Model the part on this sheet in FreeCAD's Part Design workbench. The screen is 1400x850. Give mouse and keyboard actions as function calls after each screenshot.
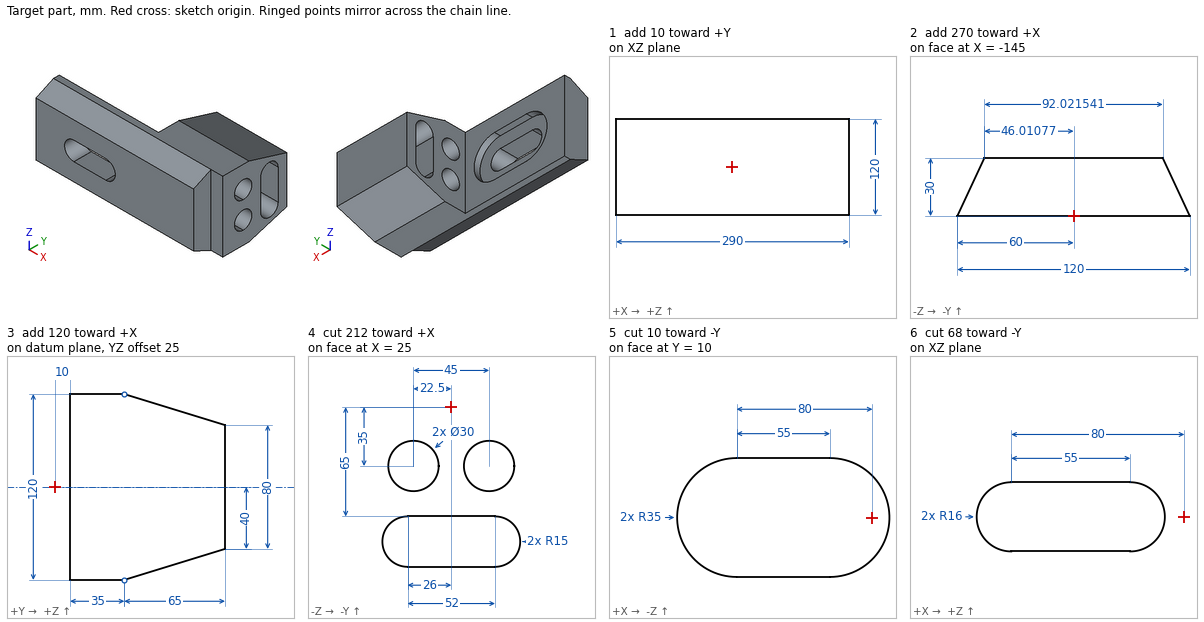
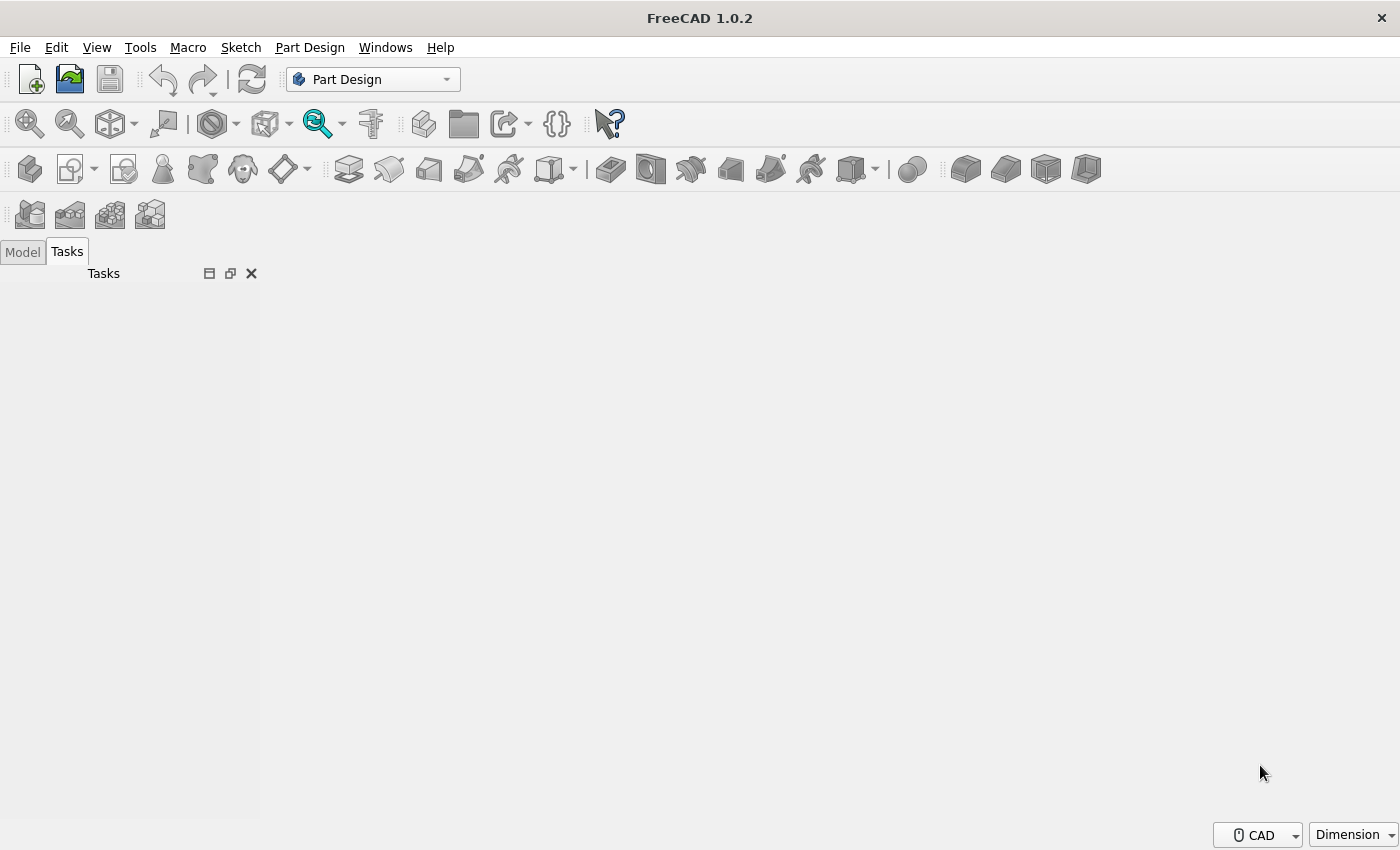
key(ctrl+n)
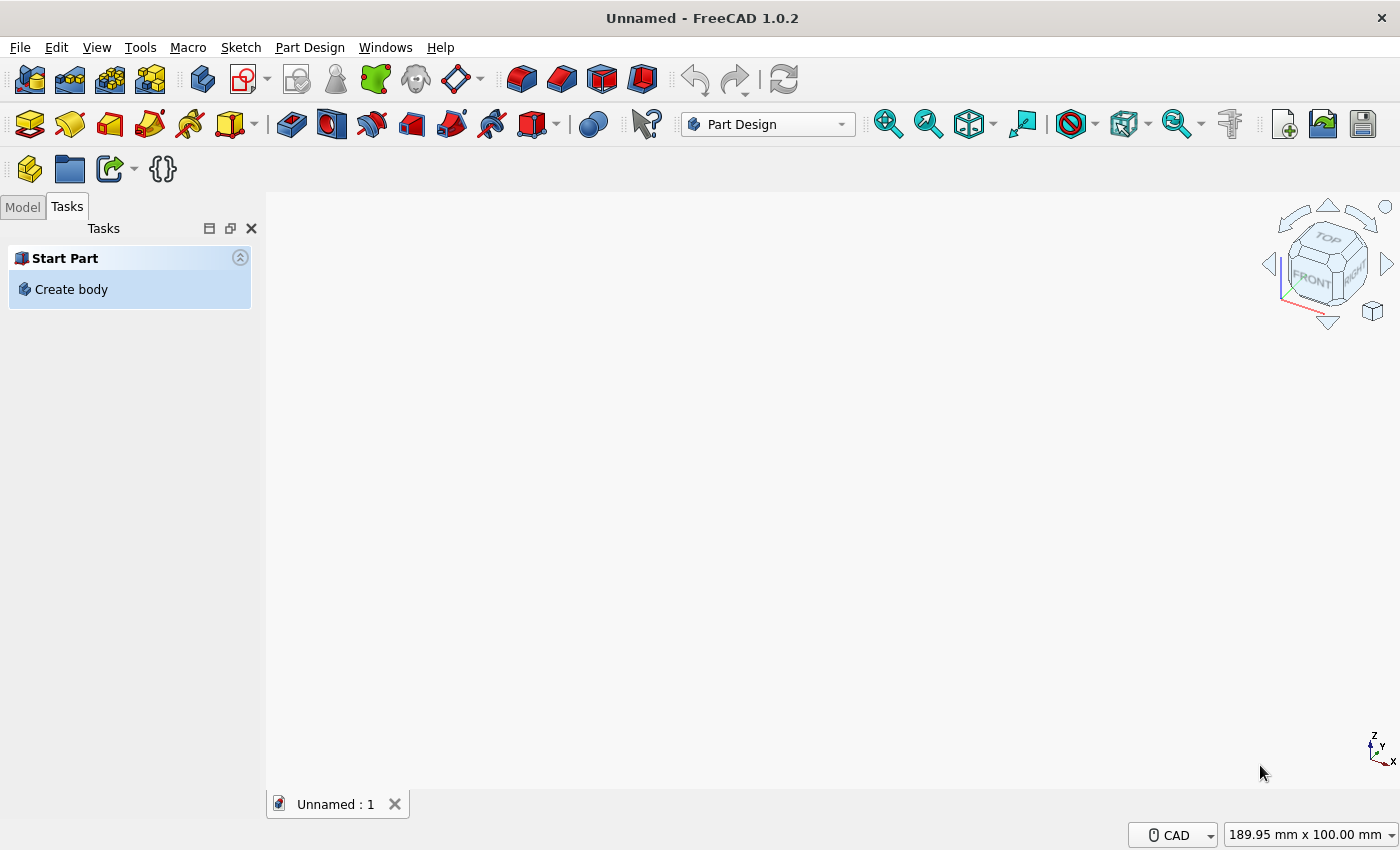
click(244, 80)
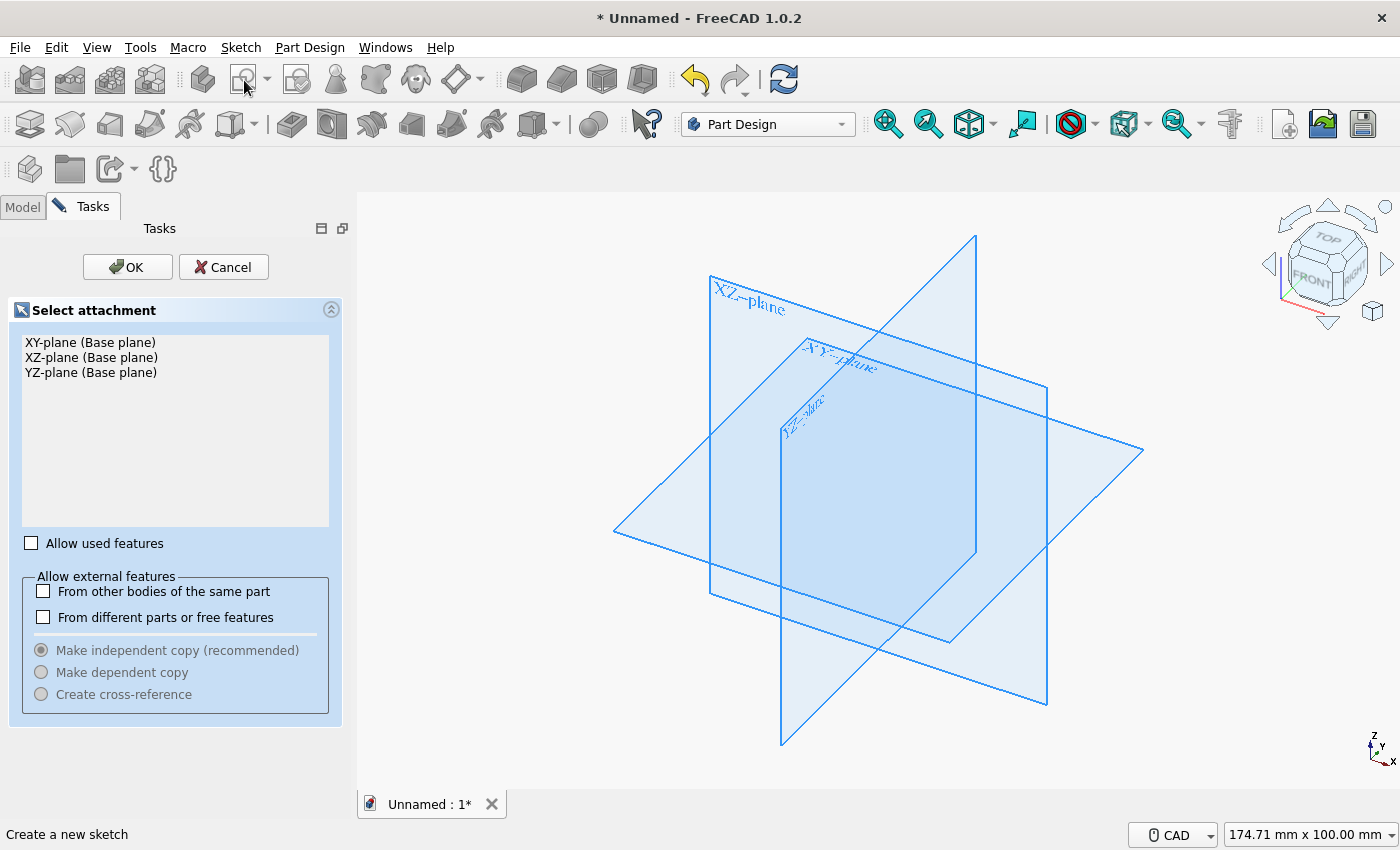
click(82, 358)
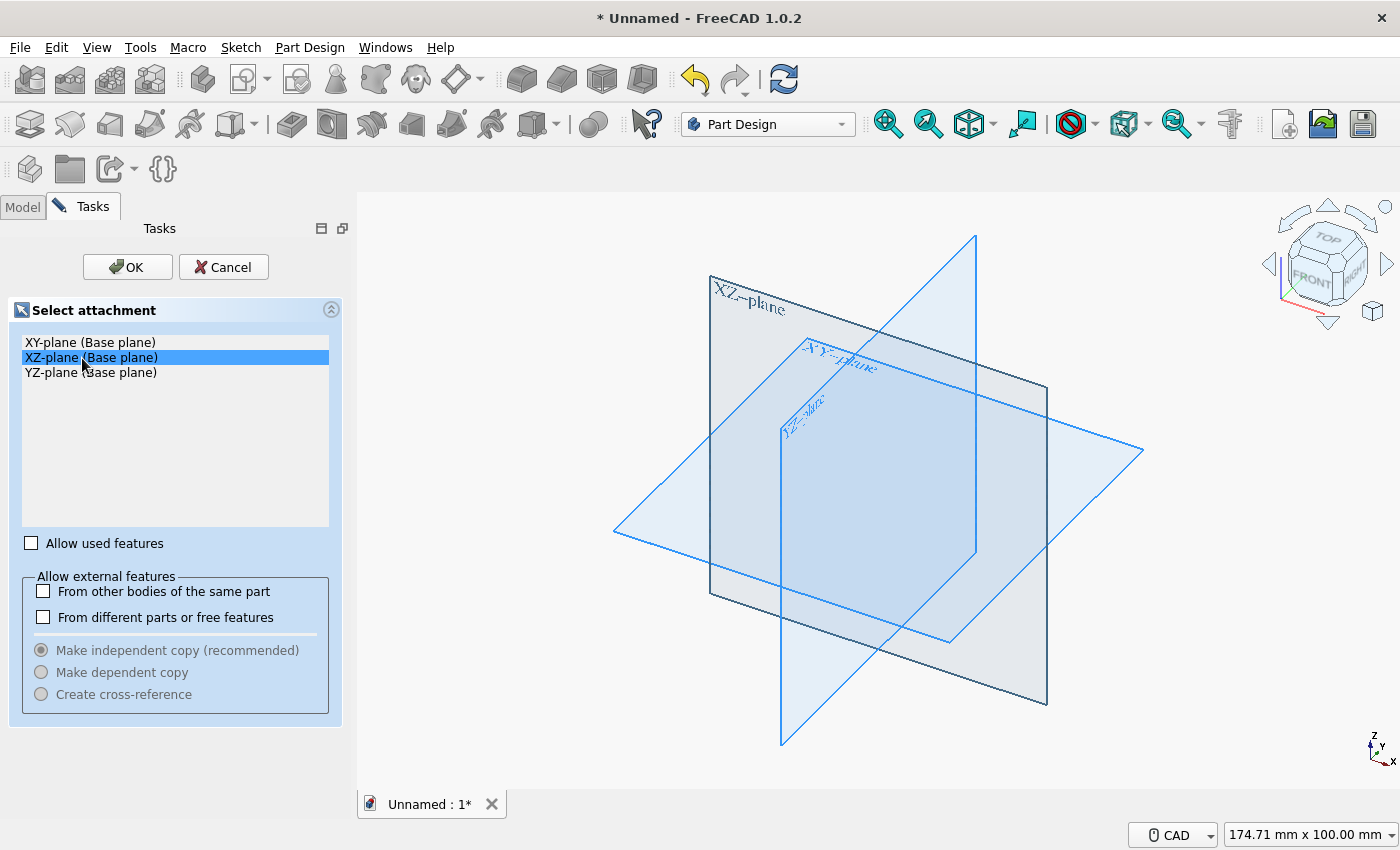
click(128, 267)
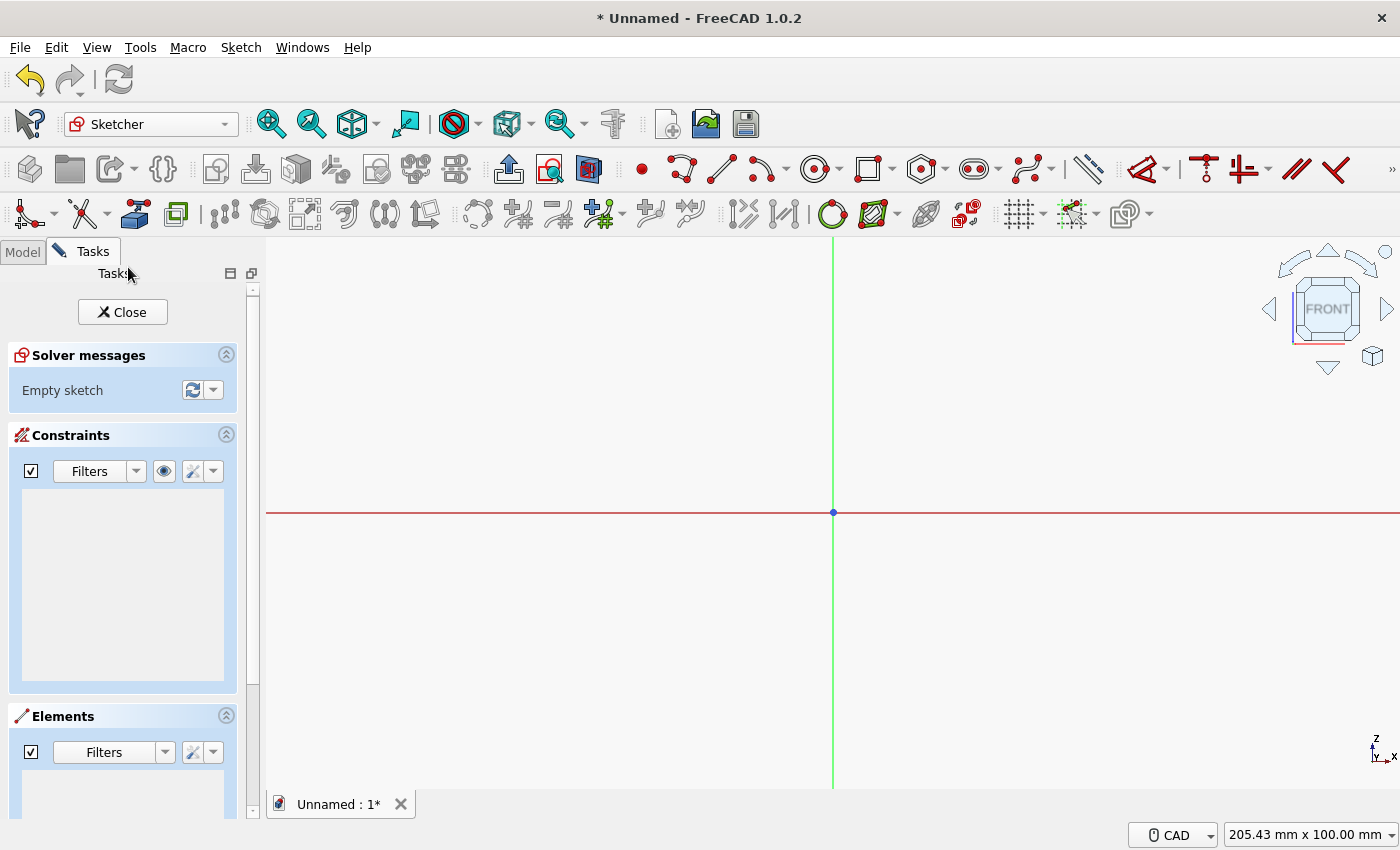
scroll(709, 513, down, 4)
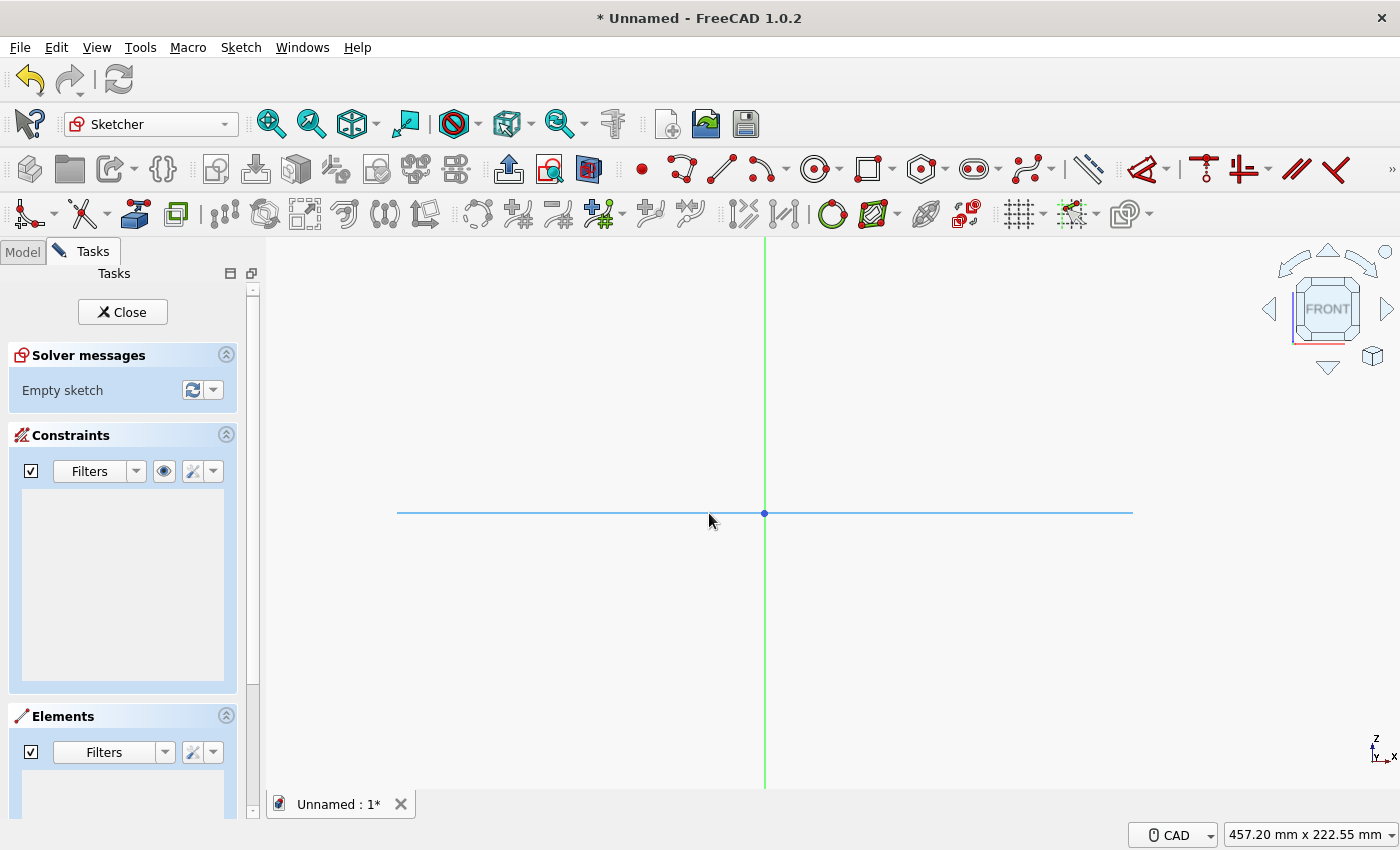
key(g)
key(v)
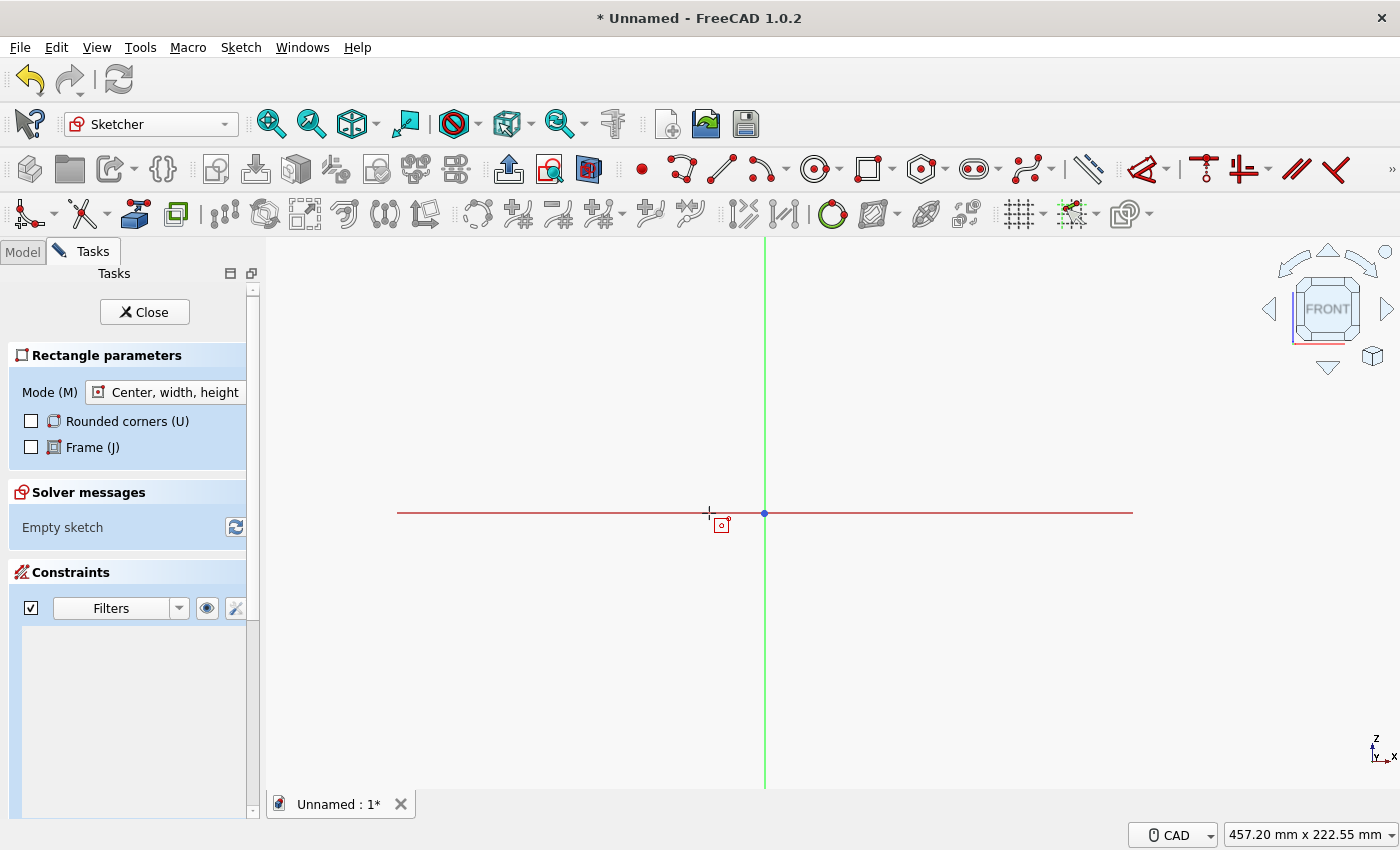
click(765, 513)
click(1125, 364)
key(Escape)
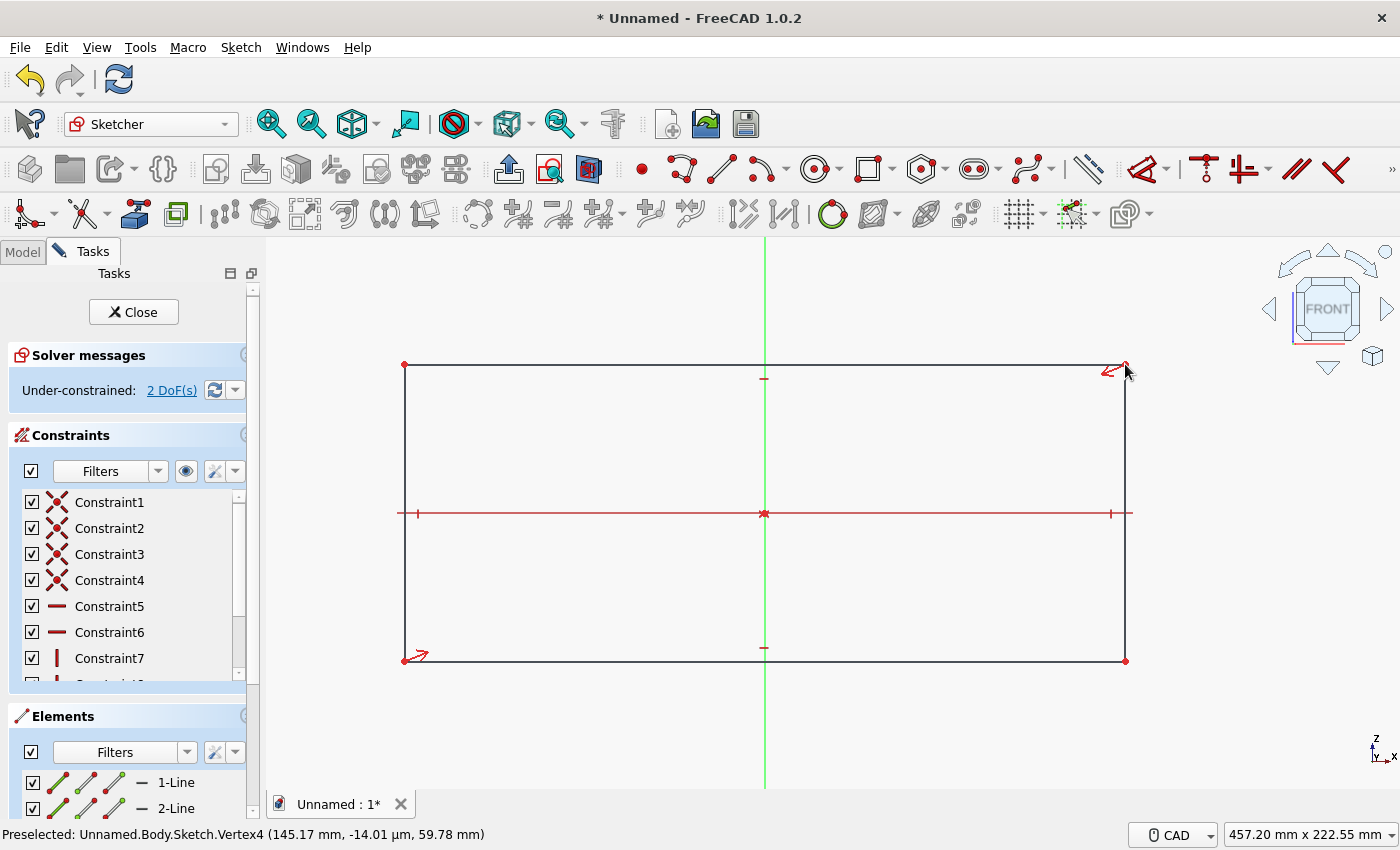
click(1142, 170)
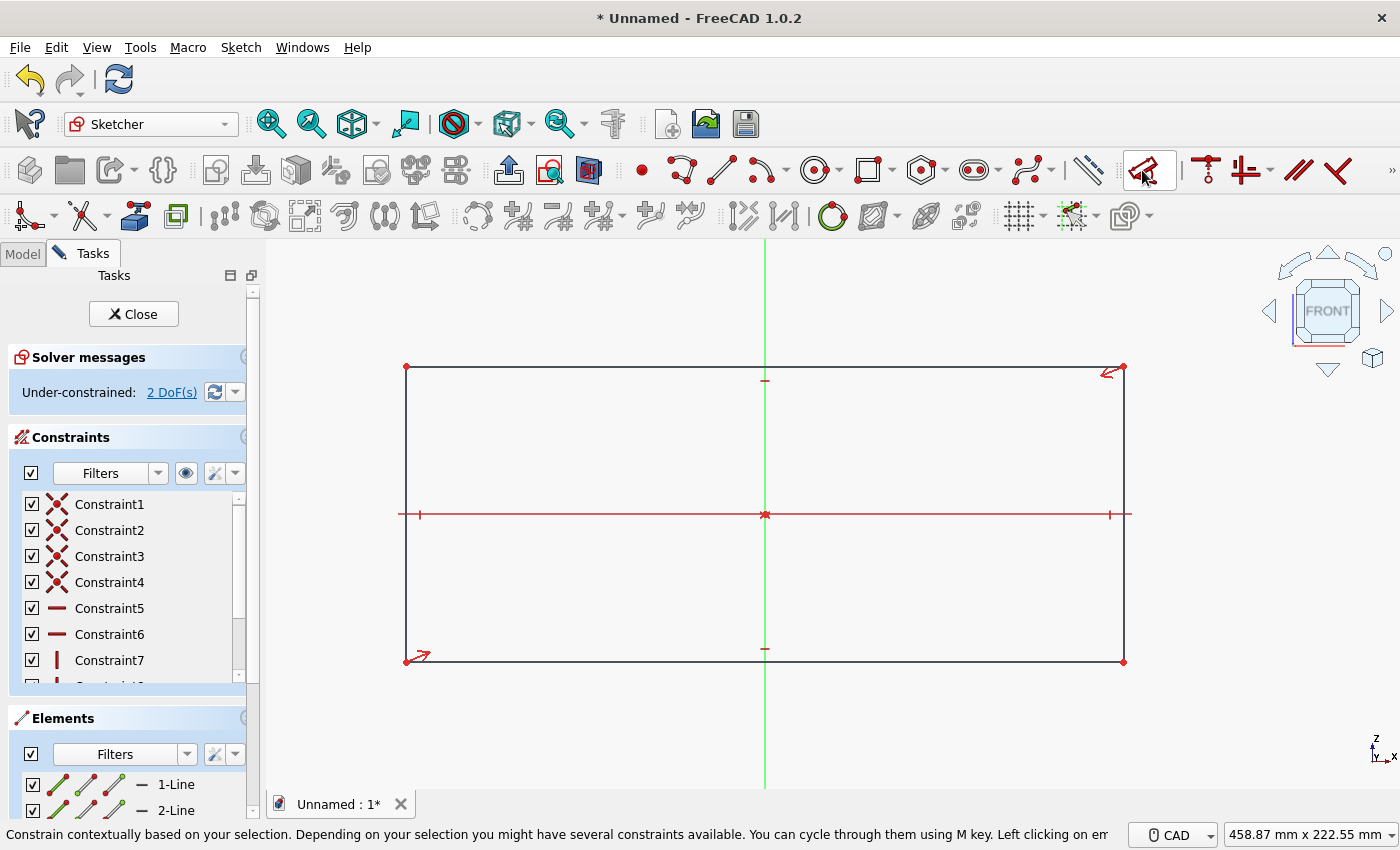
click(622, 662)
click(600, 696)